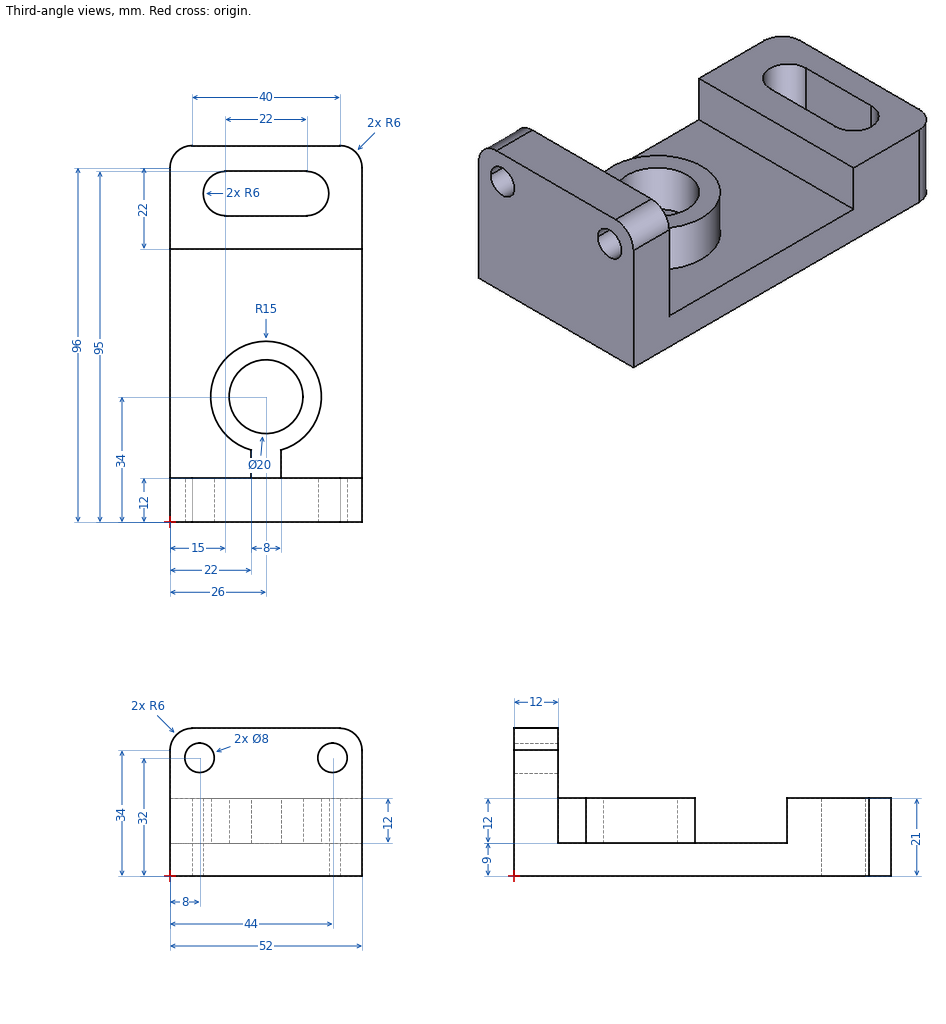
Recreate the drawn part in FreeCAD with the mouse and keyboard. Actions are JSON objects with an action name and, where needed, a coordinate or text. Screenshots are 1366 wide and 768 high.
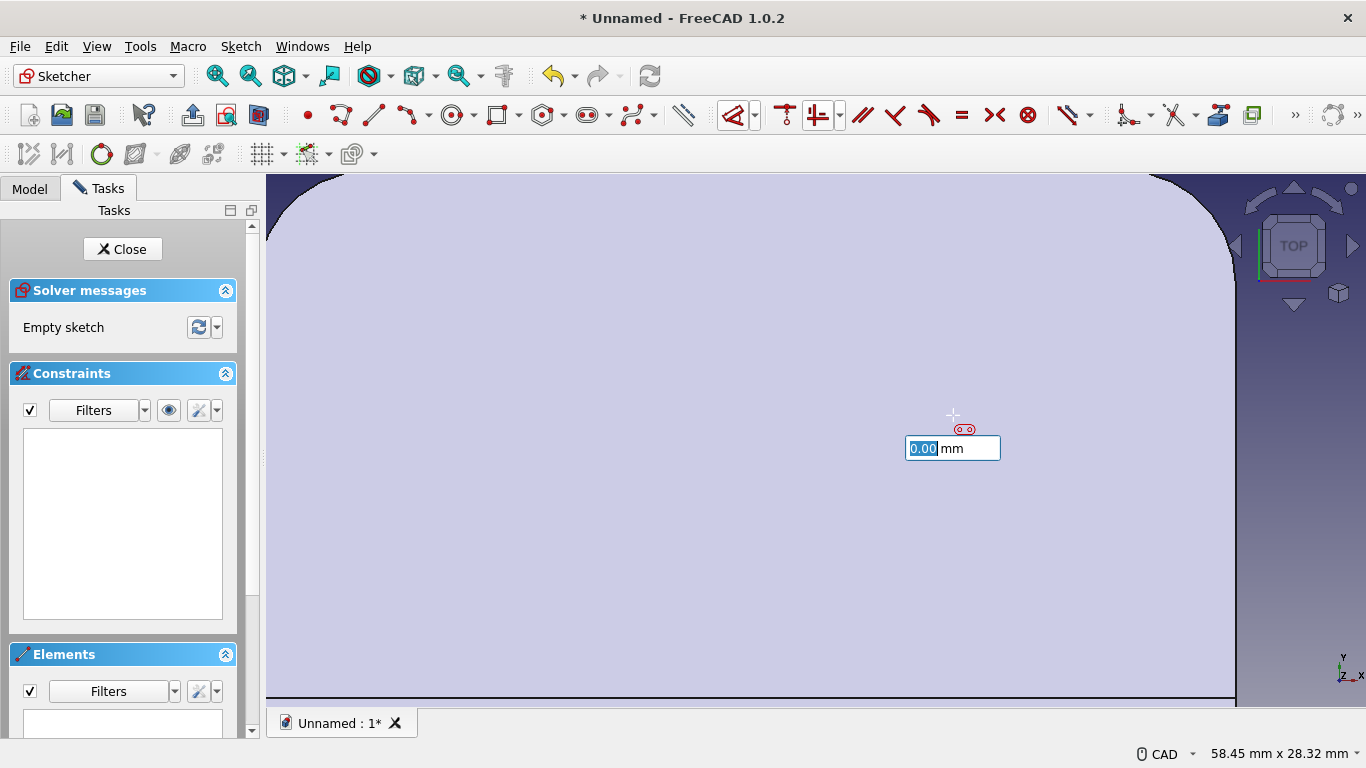
{"action": "left_click", "coordinate": [746, 528]}
{"action": "key", "text": "Escape"}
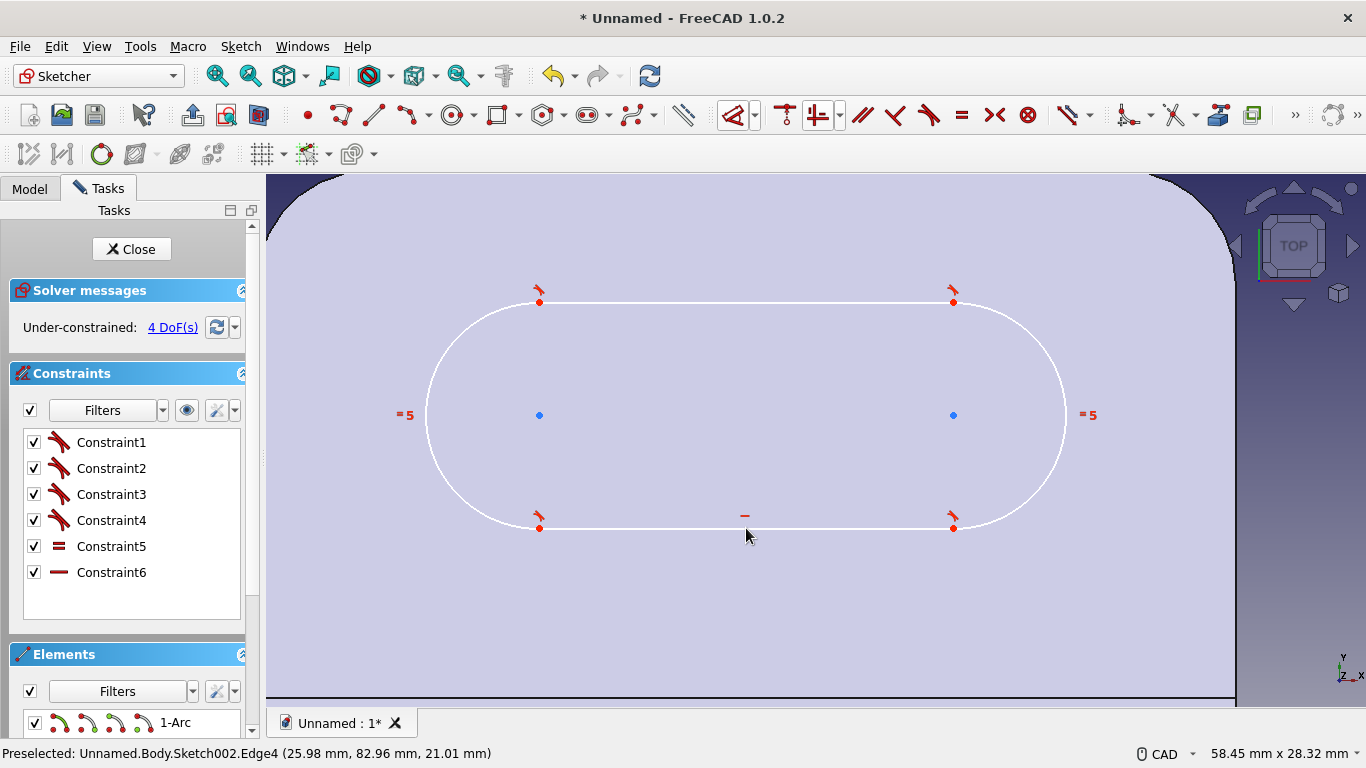
{"action": "left_click", "coordinate": [448, 350]}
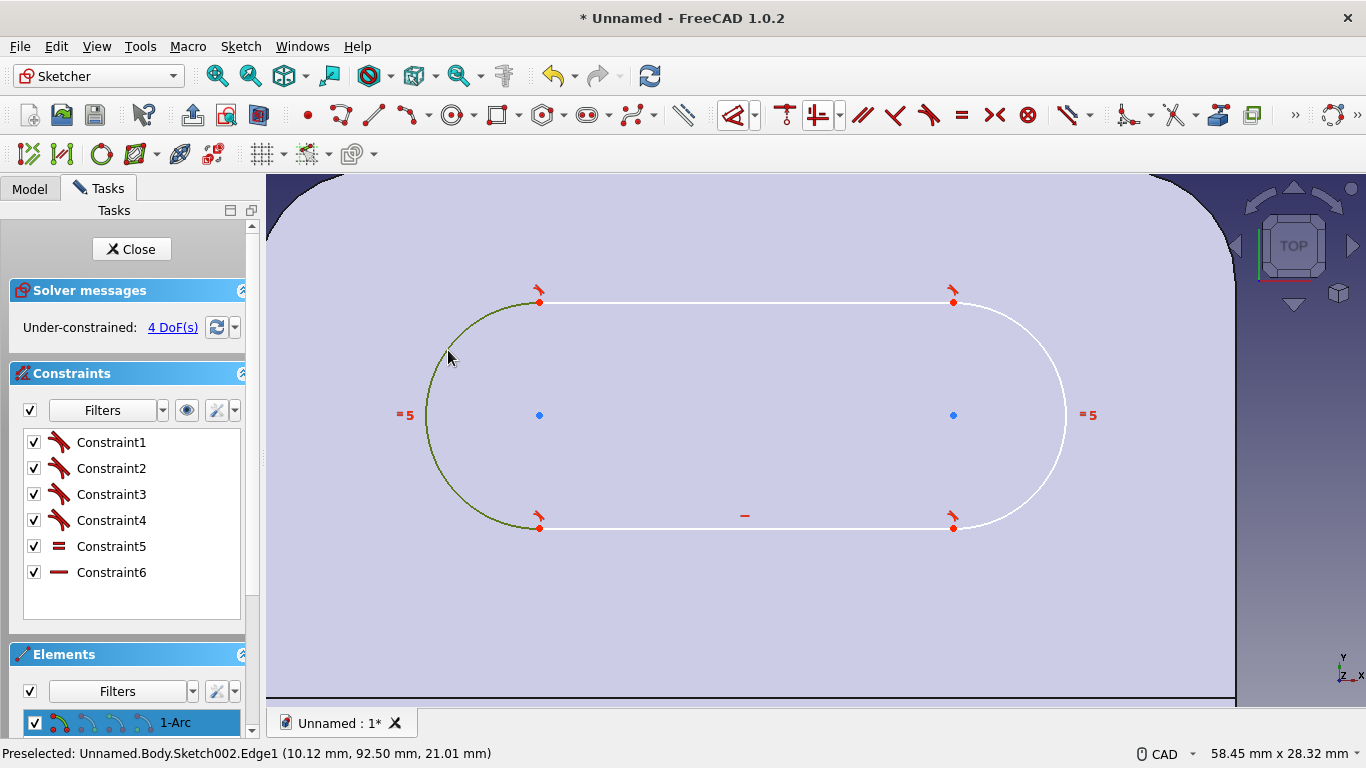
{"action": "left_click", "coordinate": [754, 116]}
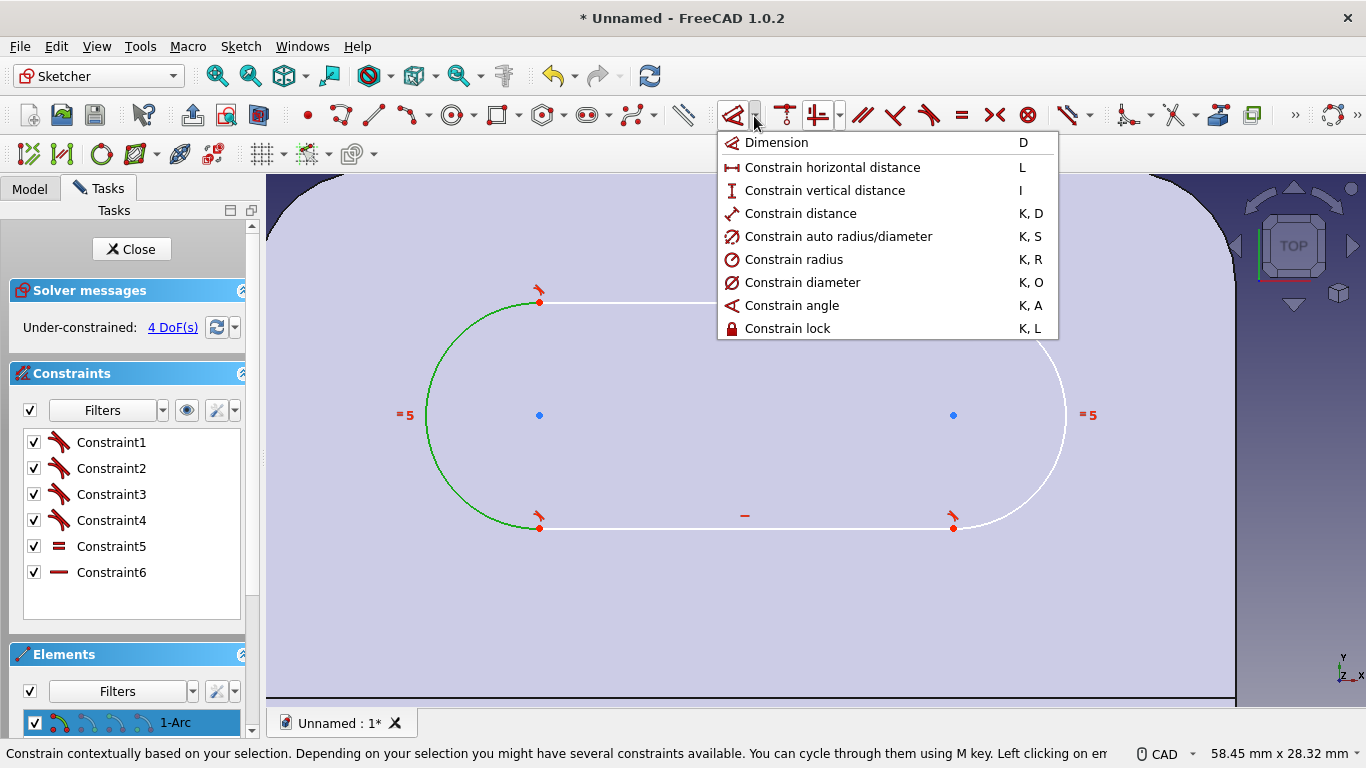
{"action": "left_click", "coordinate": [888, 260]}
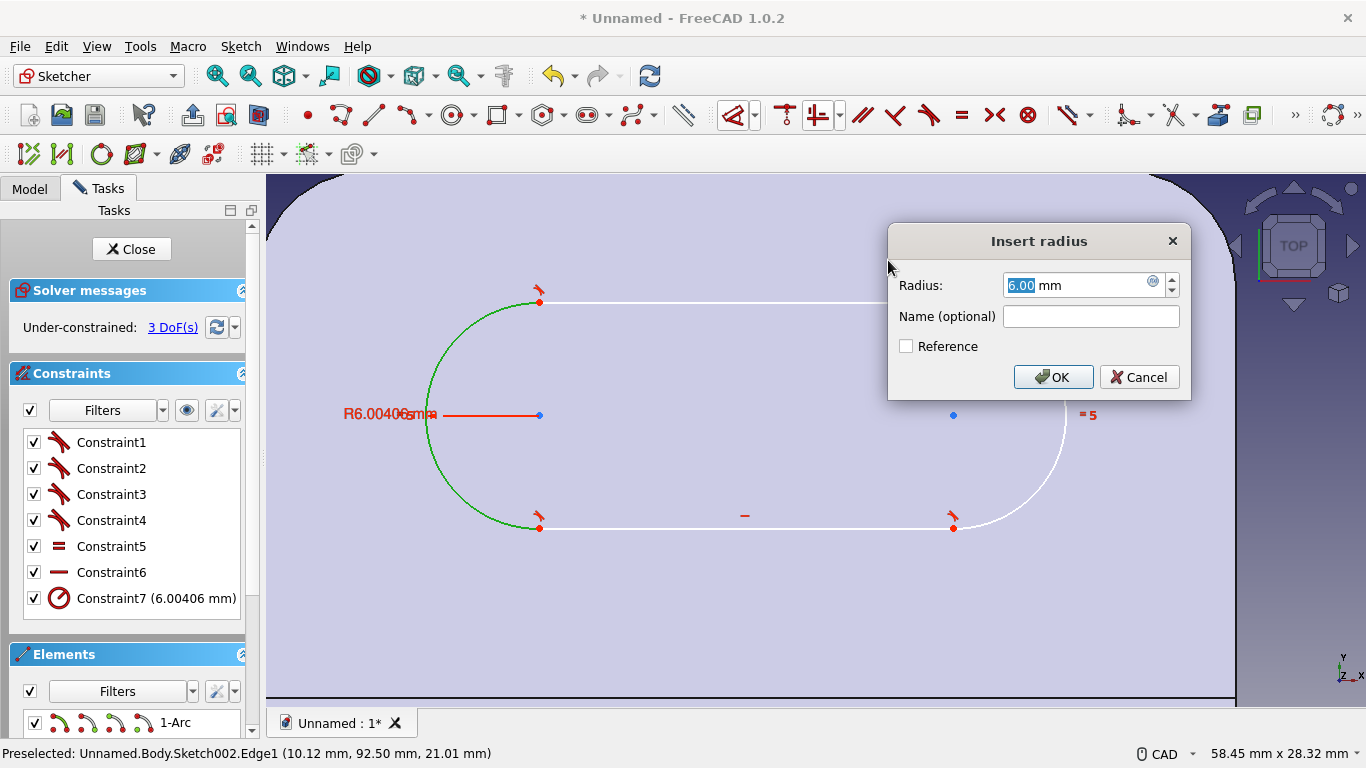
{"action": "type", "text": "6"}
{"action": "key", "text": "Return"}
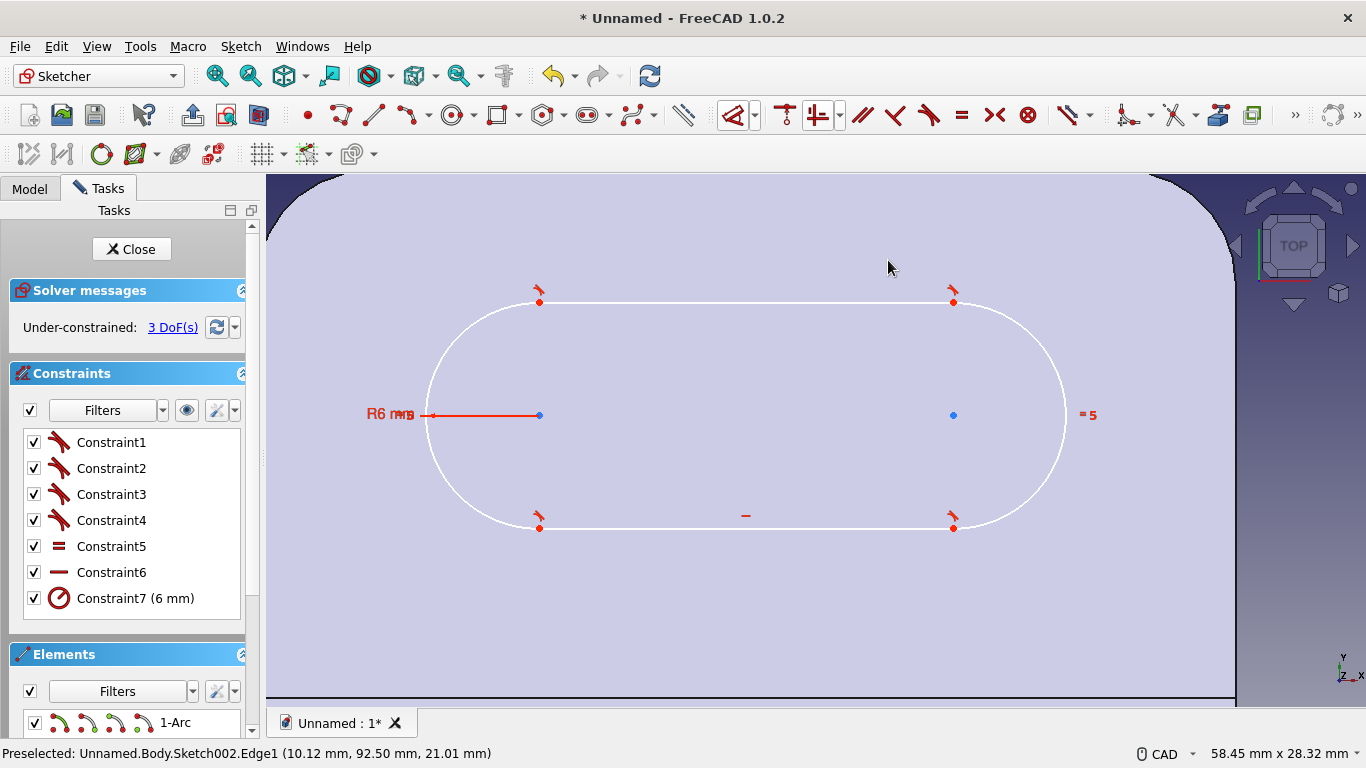
{"action": "left_click", "coordinate": [663, 303]}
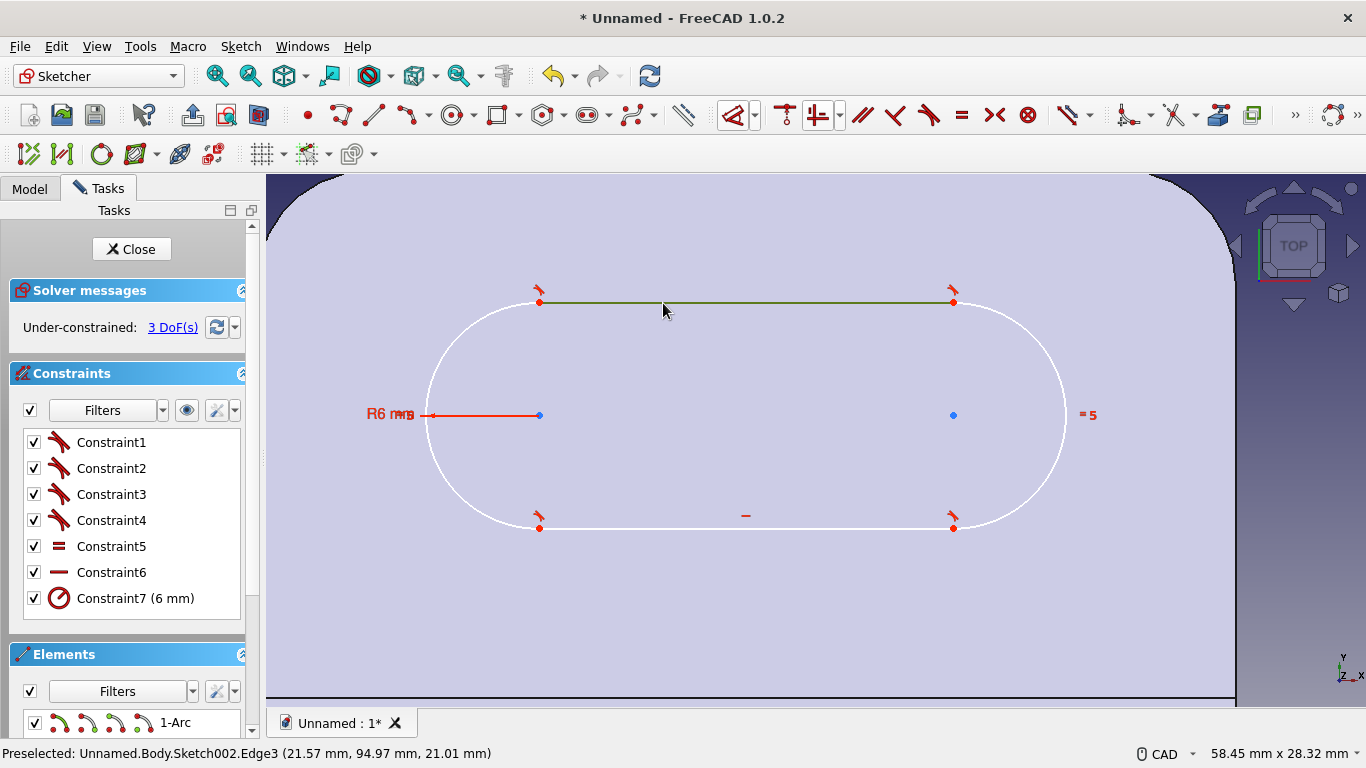
{"action": "left_click", "coordinate": [754, 116]}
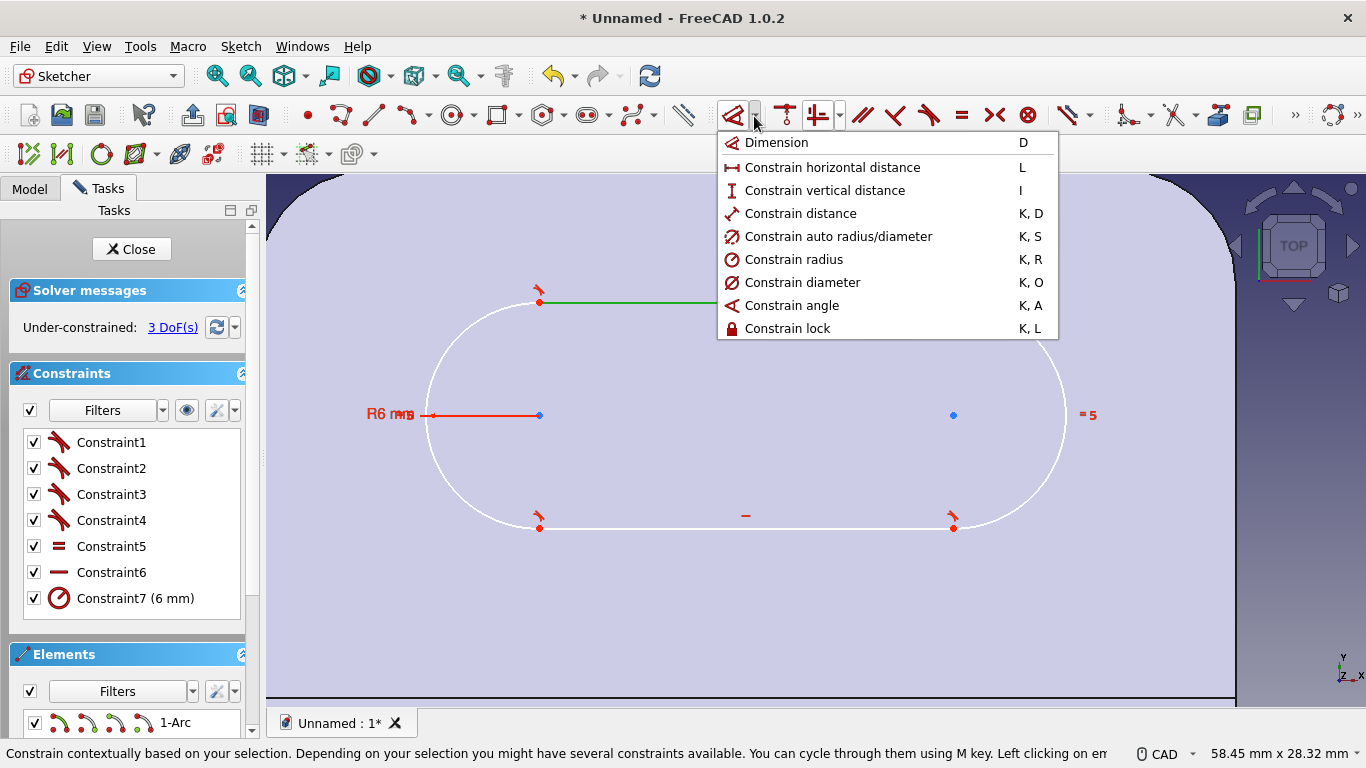
{"action": "left_click", "coordinate": [888, 168]}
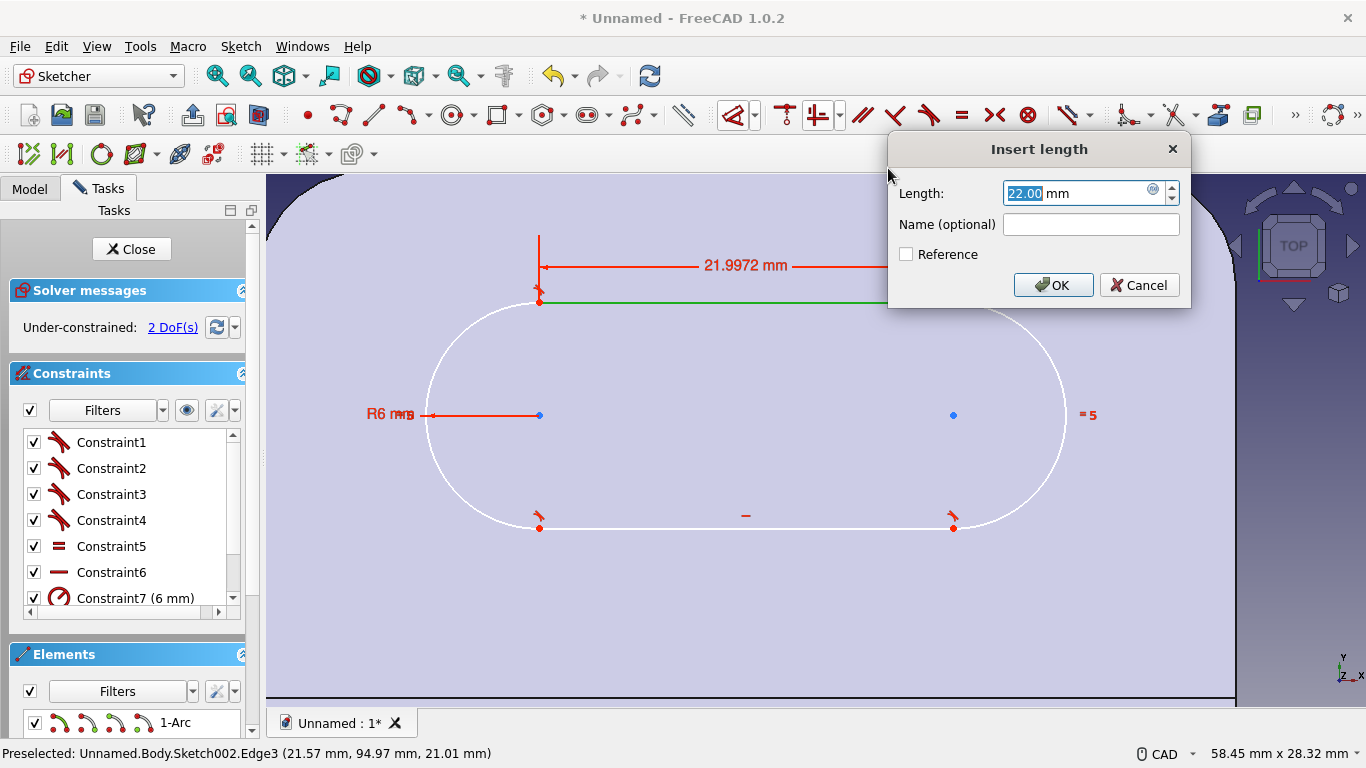
{"action": "type", "text": "22"}
{"action": "key", "text": "Return"}